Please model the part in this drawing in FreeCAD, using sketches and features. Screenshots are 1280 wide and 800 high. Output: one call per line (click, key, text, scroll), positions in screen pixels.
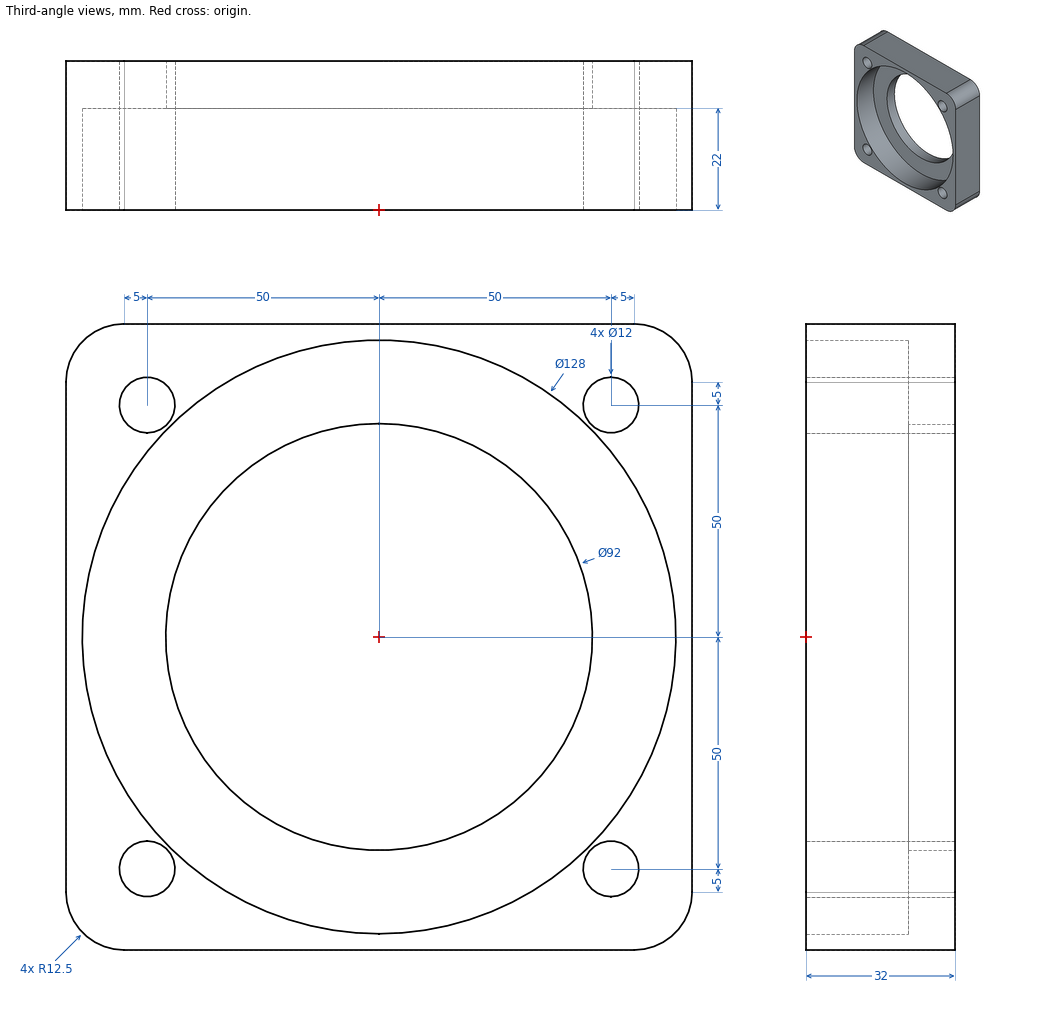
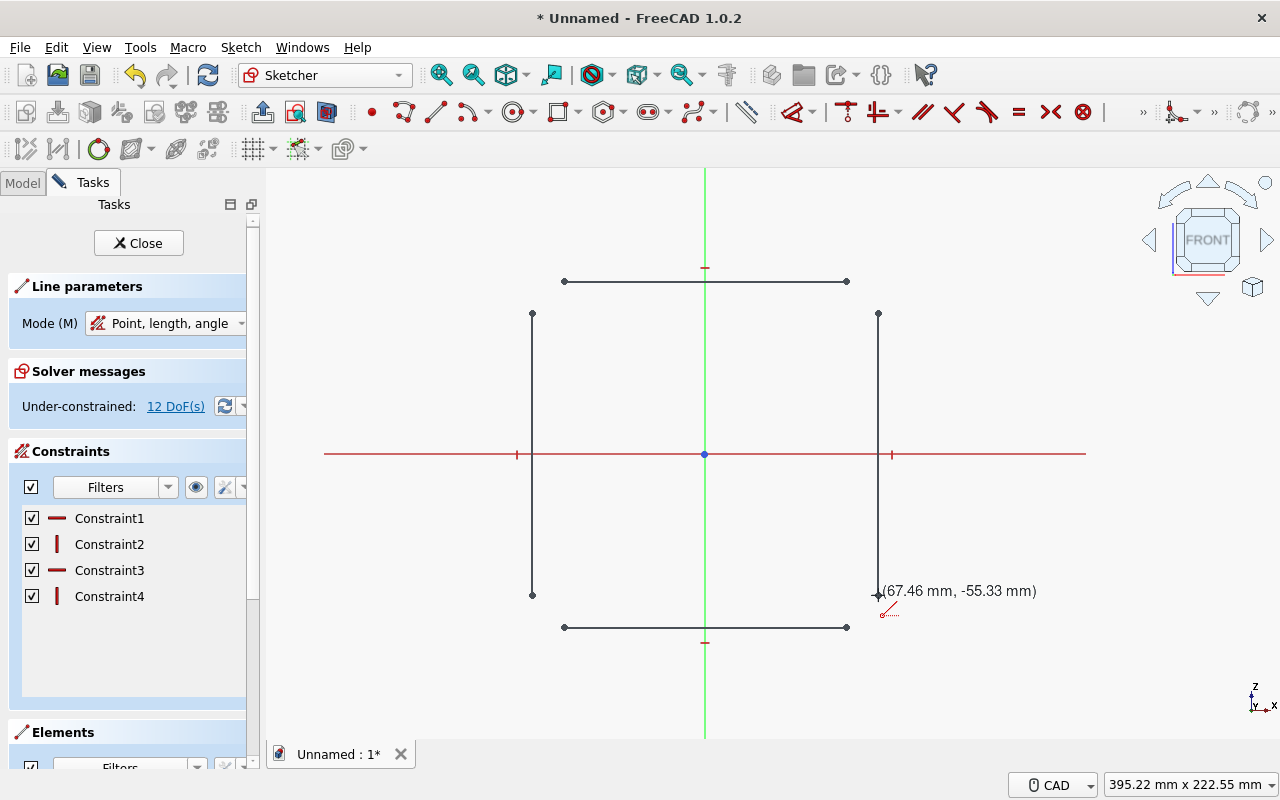
click(490, 112)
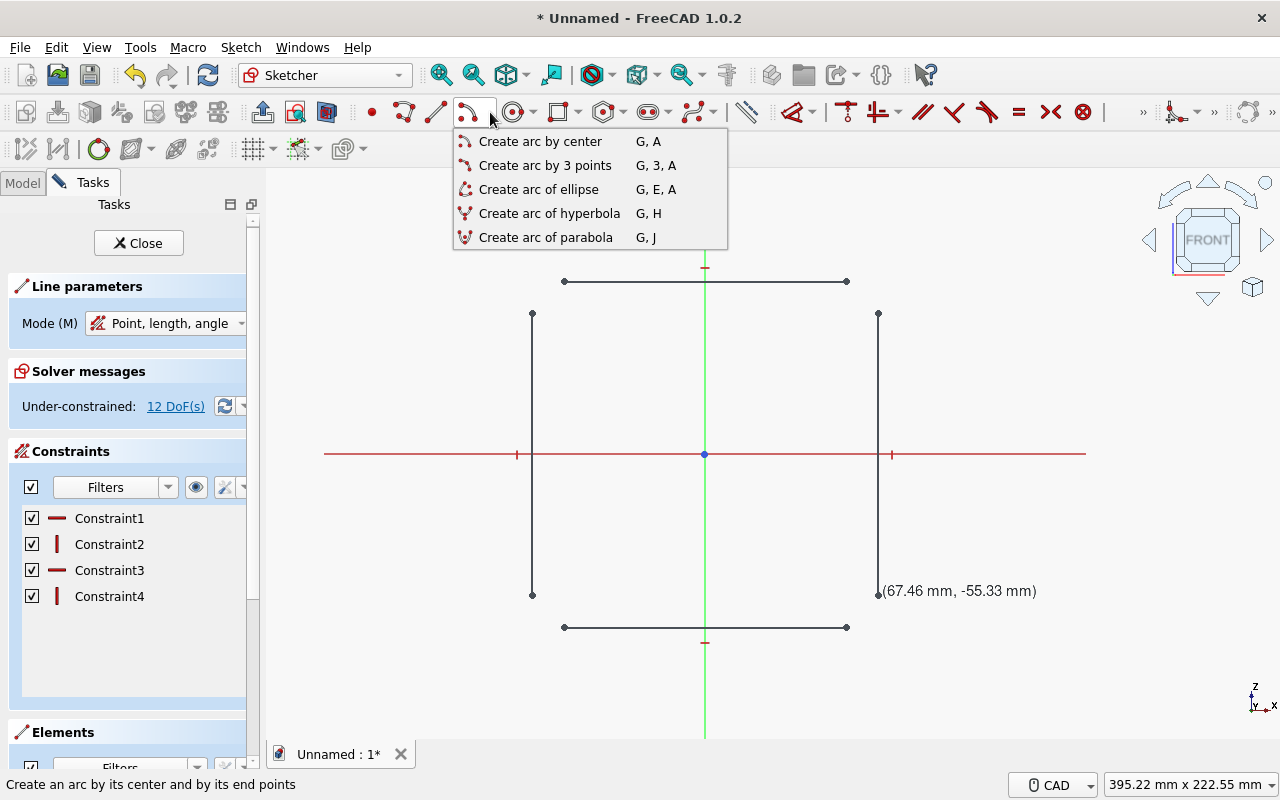
click(590, 165)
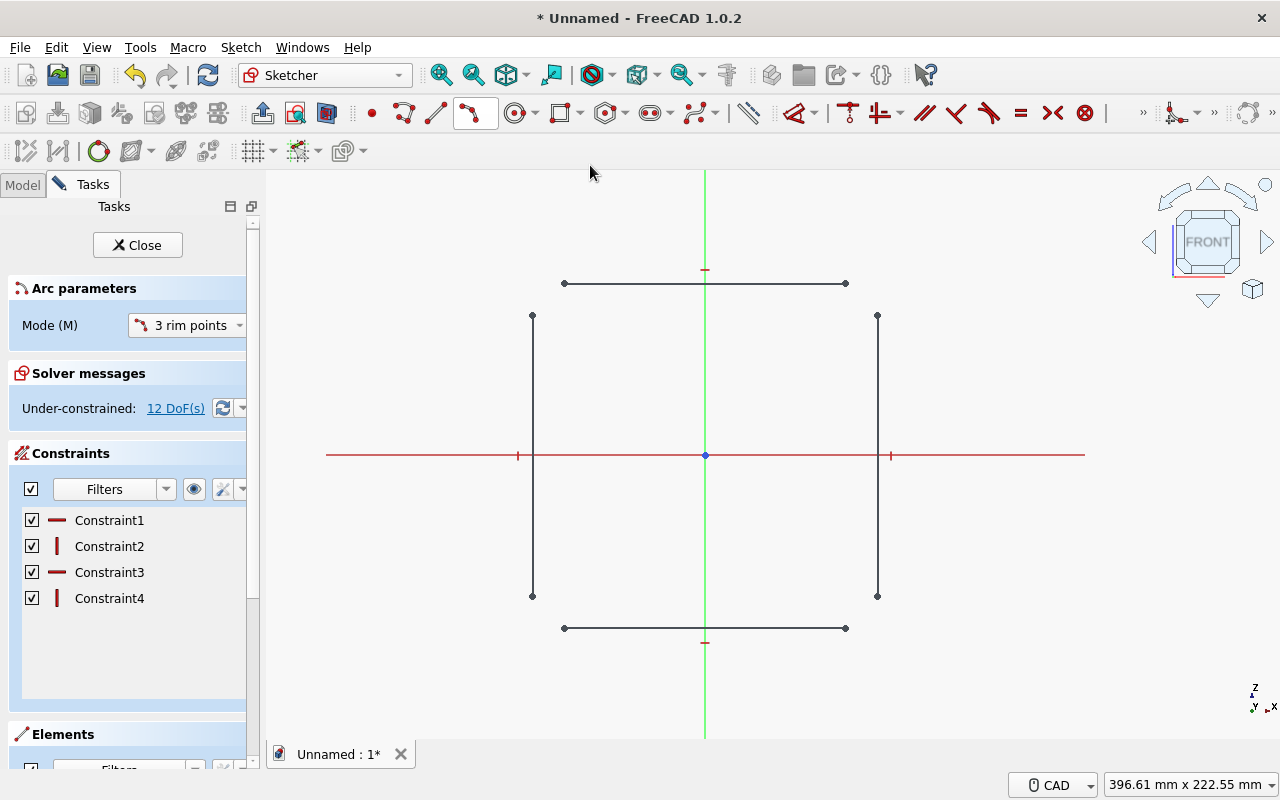
click(565, 628)
click(533, 597)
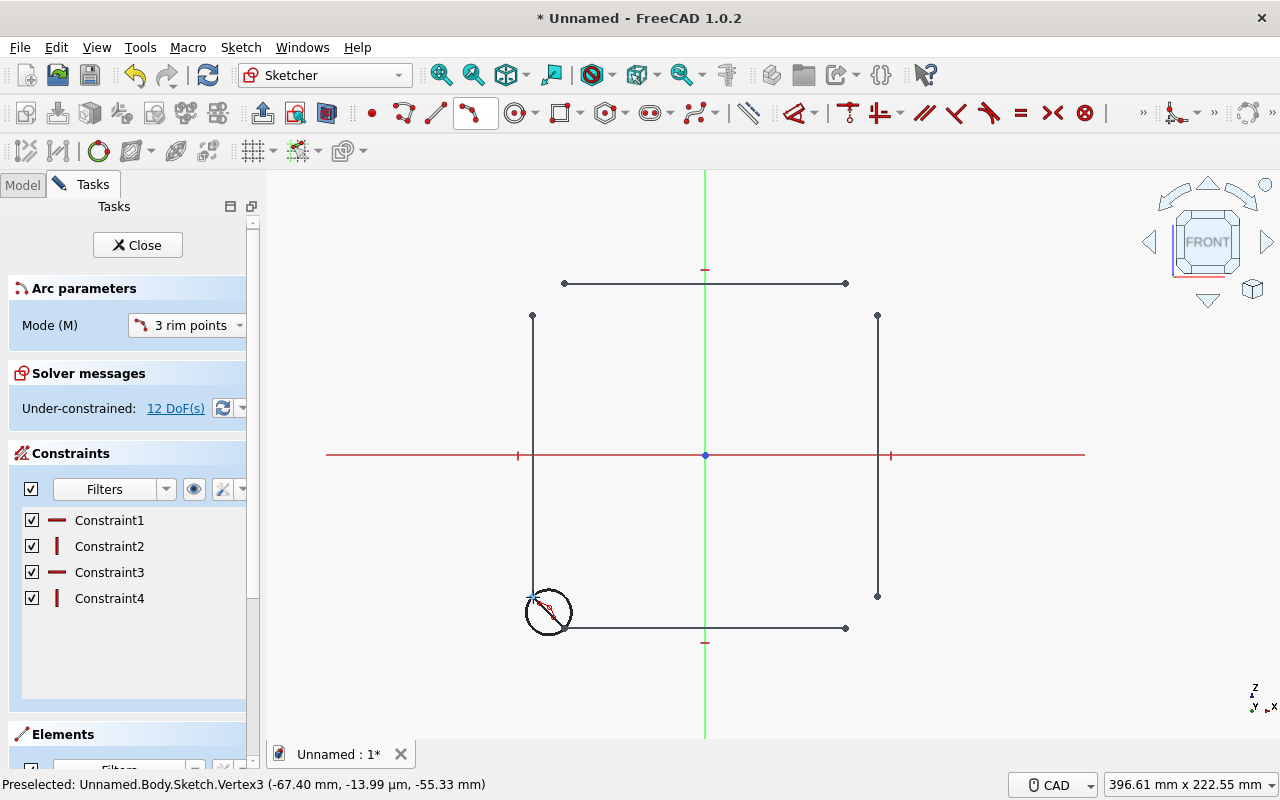
scroll(542, 618, up, 3)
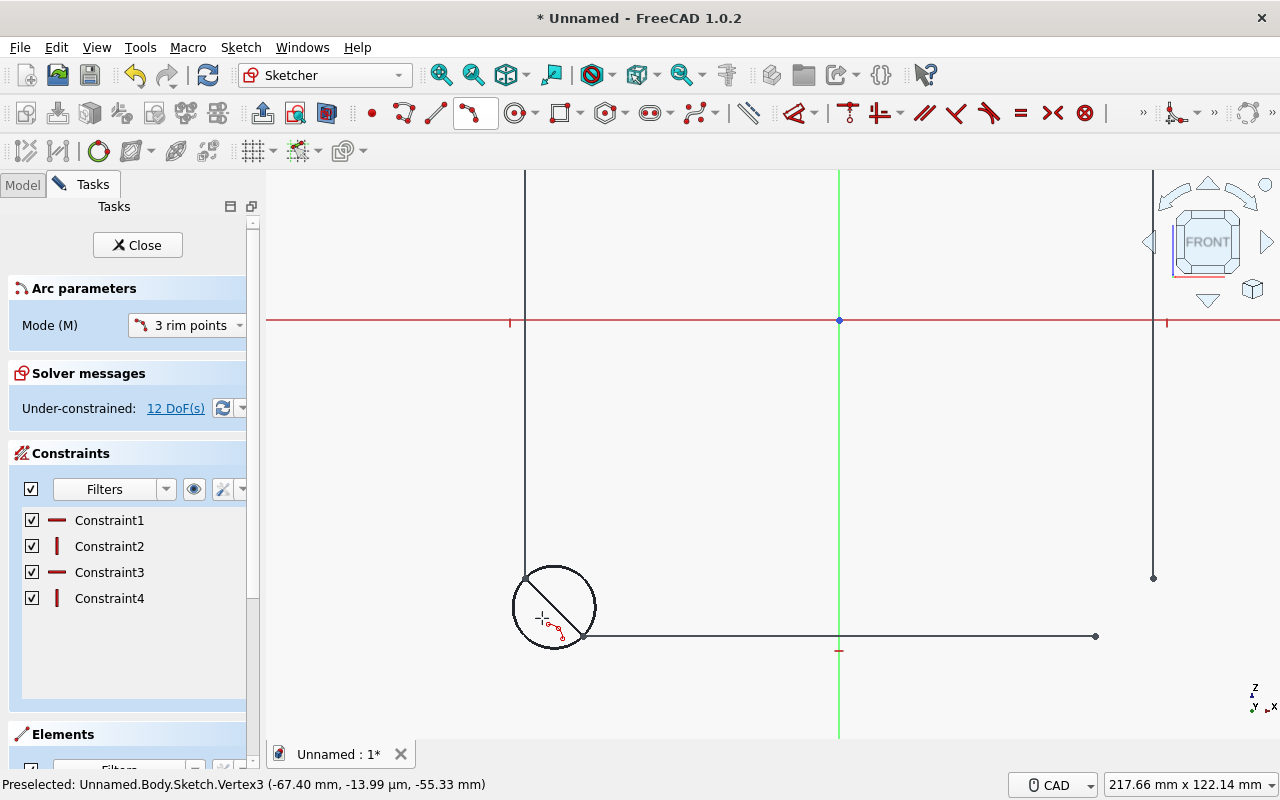
click(542, 618)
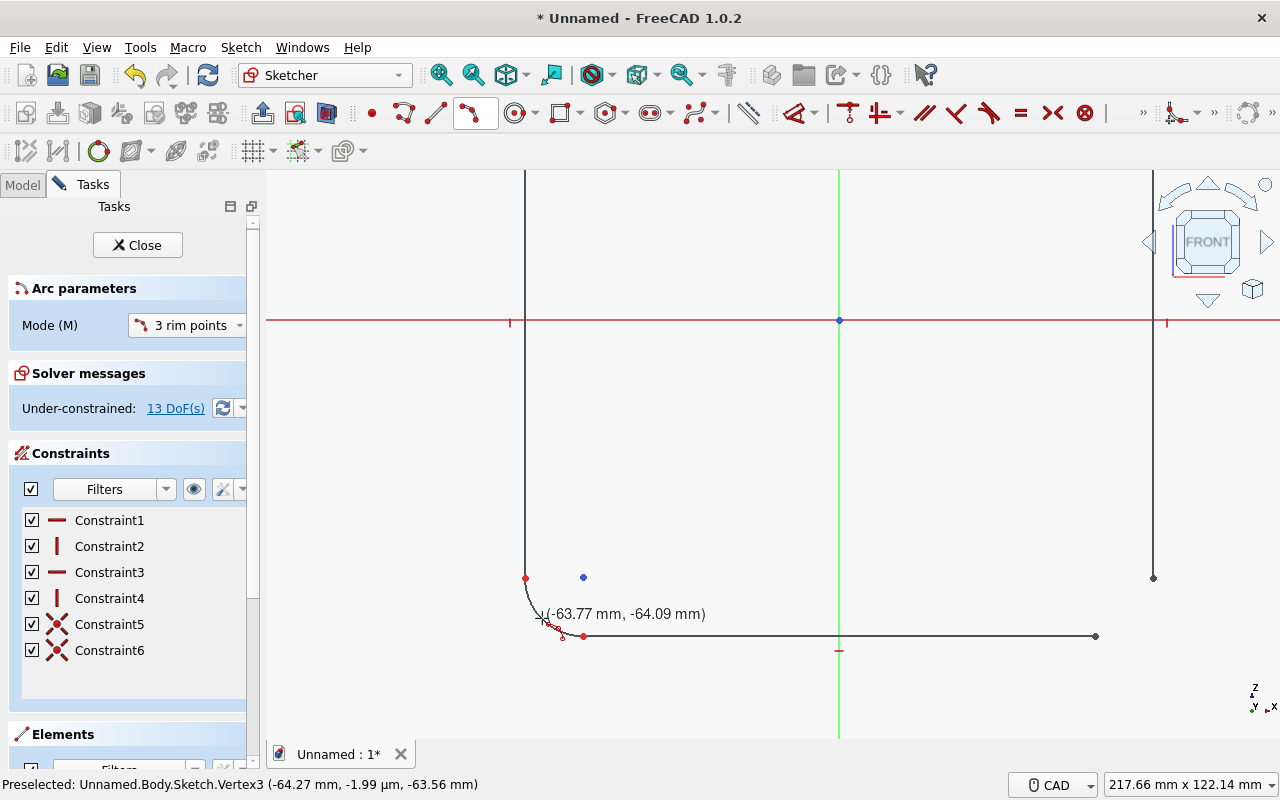
scroll(541, 618, down, 3)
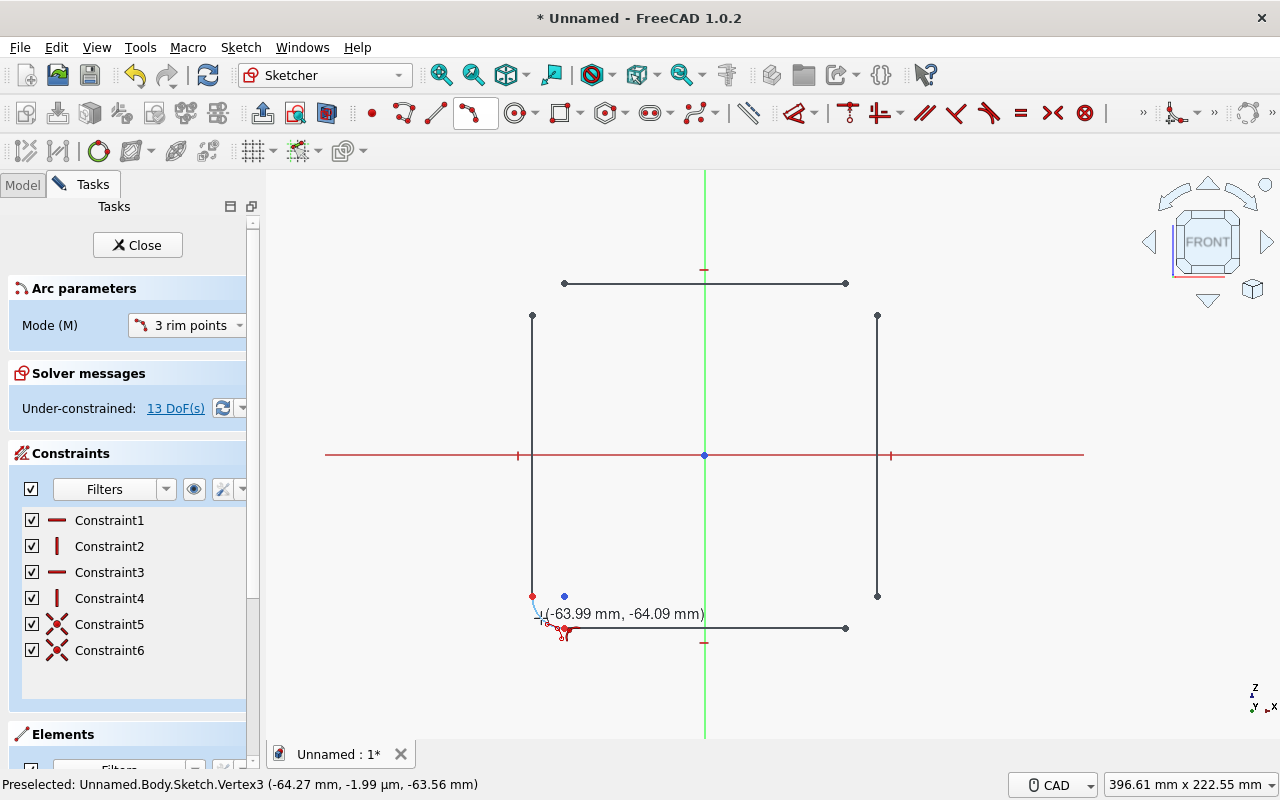
click(532, 315)
click(564, 284)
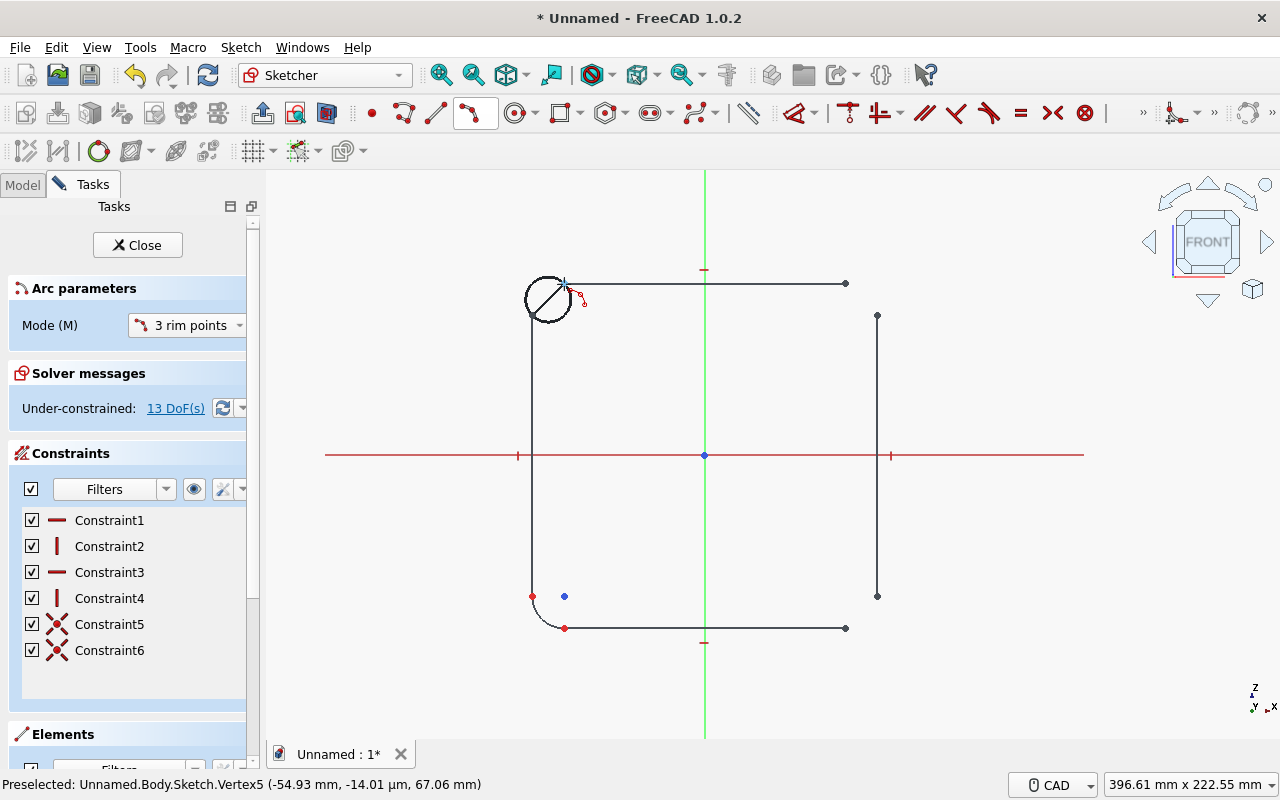
scroll(541, 292, up, 3)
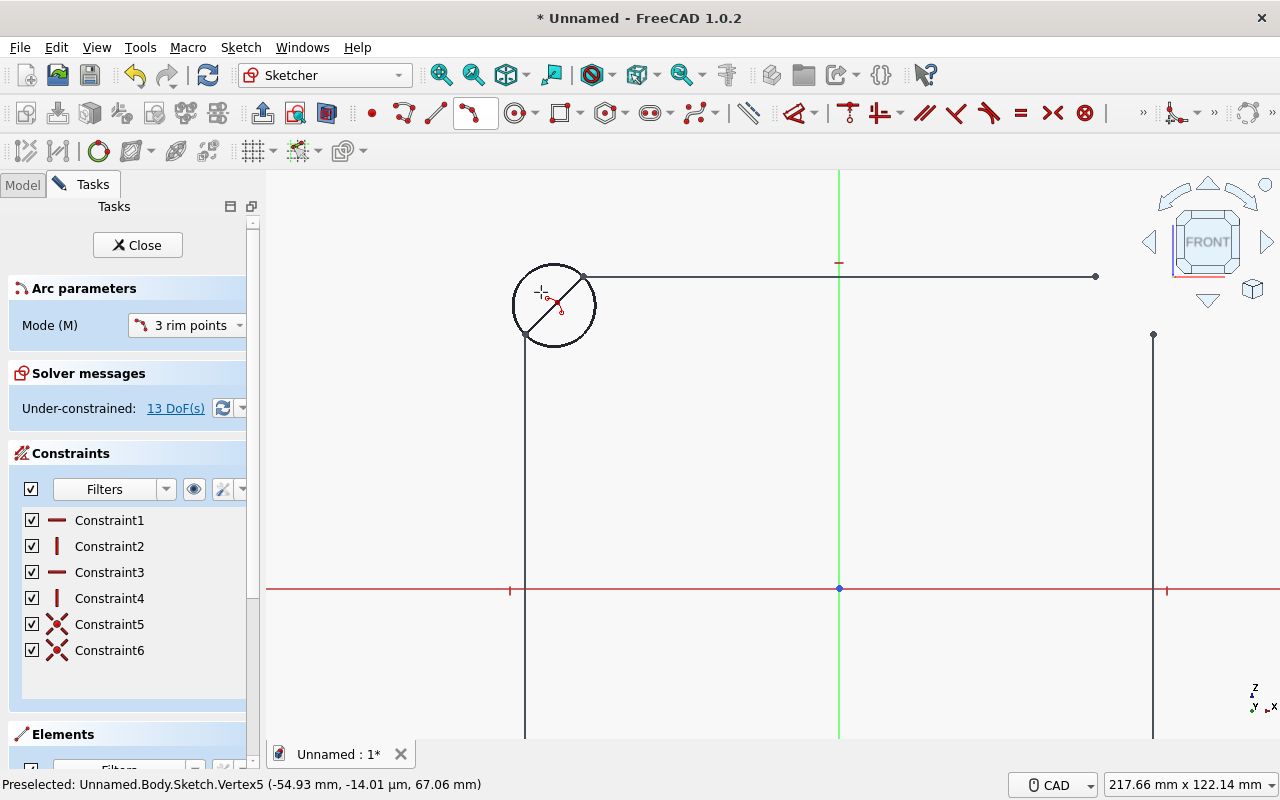
click(542, 292)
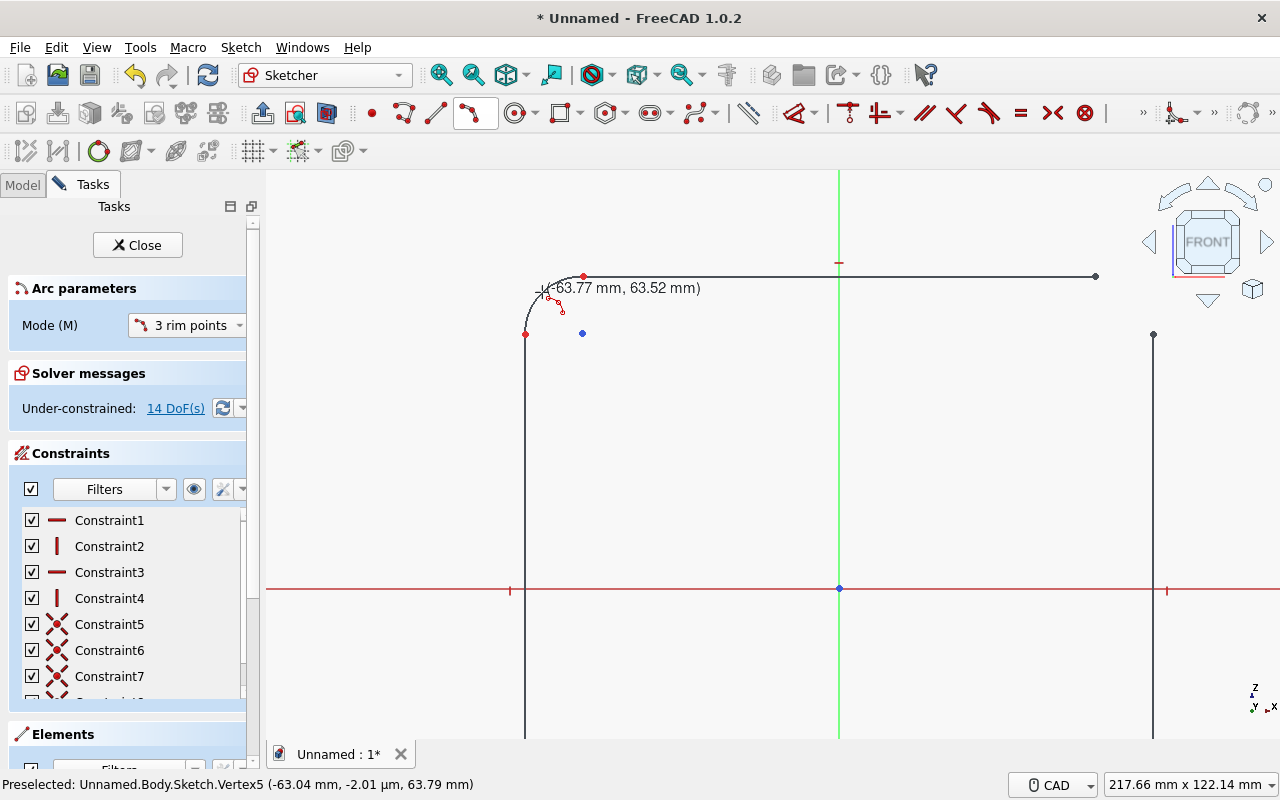
click(1095, 277)